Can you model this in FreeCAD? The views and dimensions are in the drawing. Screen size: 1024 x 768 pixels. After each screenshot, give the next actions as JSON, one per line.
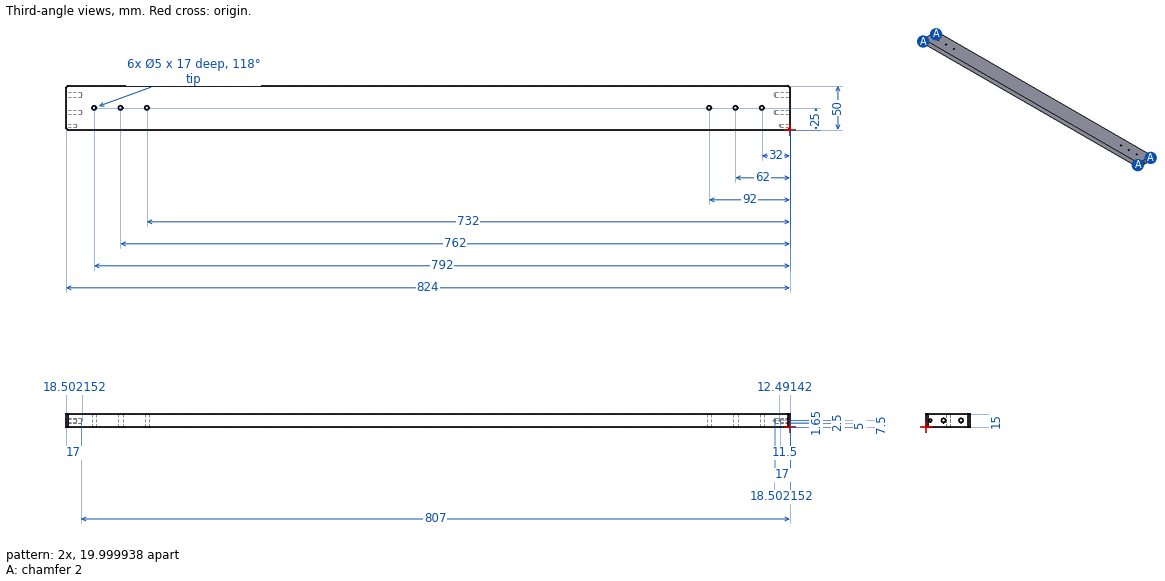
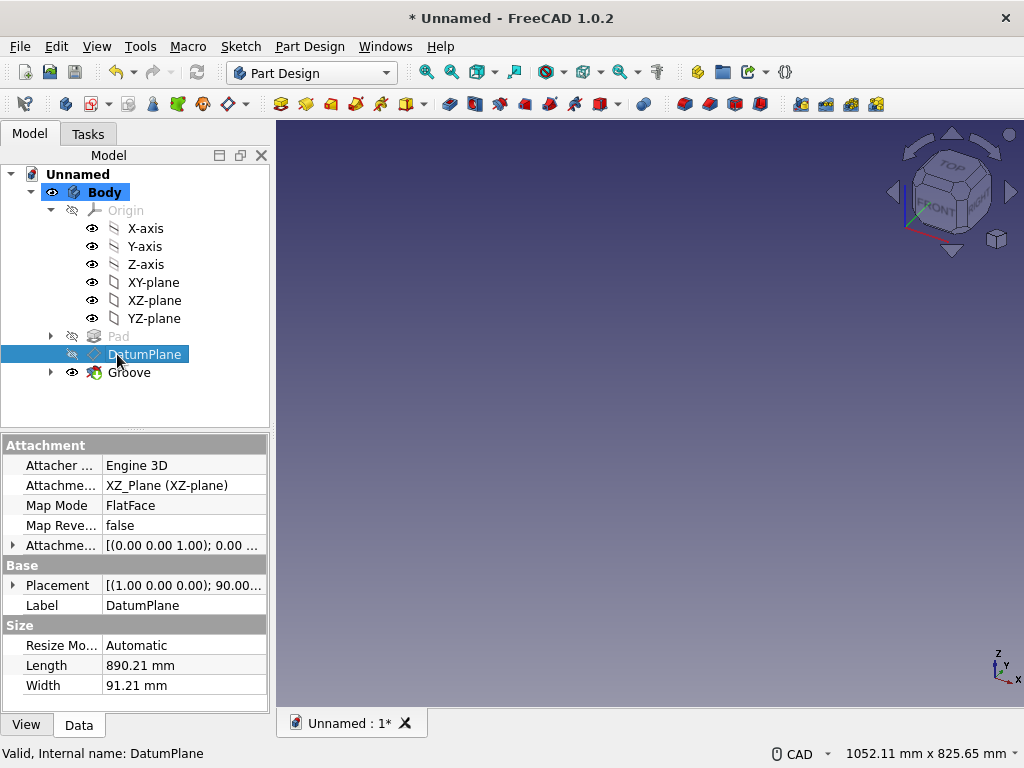
{"action": "left_click", "coordinate": [427, 72]}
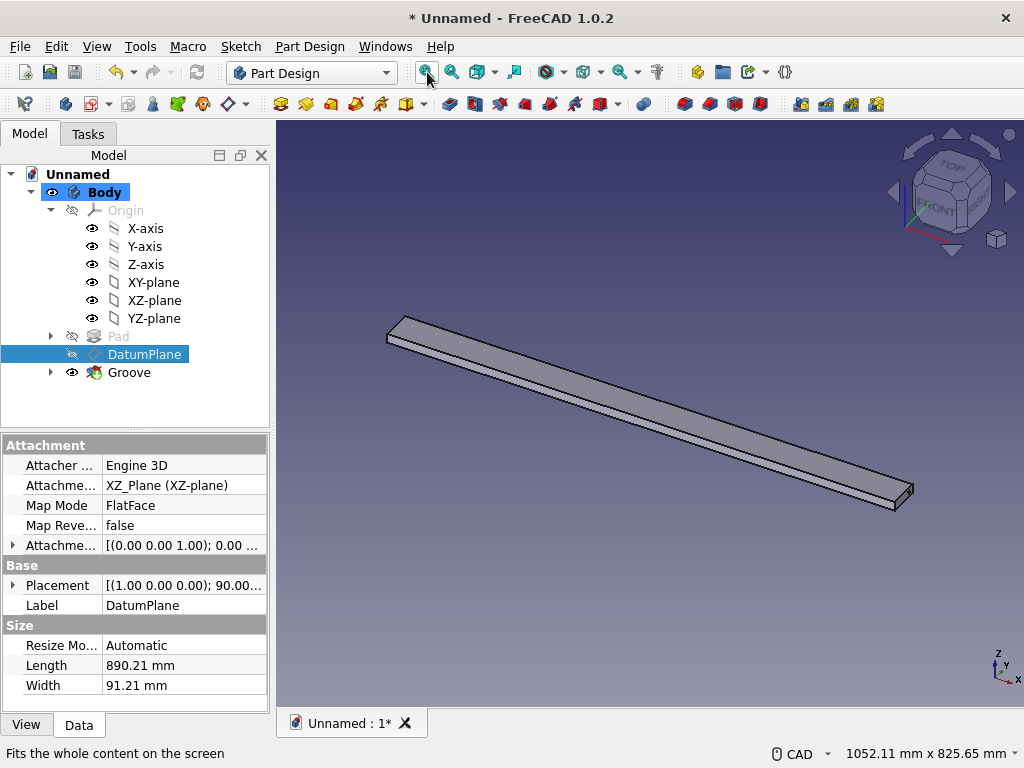
{"action": "left_click", "coordinate": [117, 372]}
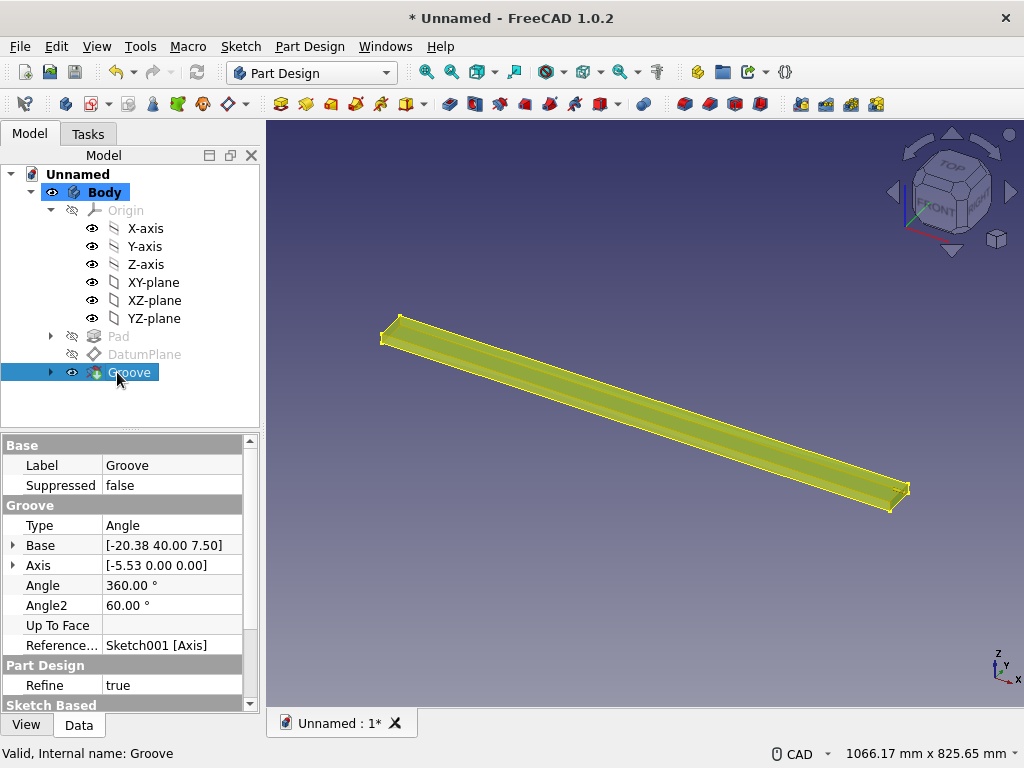
{"action": "left_click", "coordinate": [826, 104]}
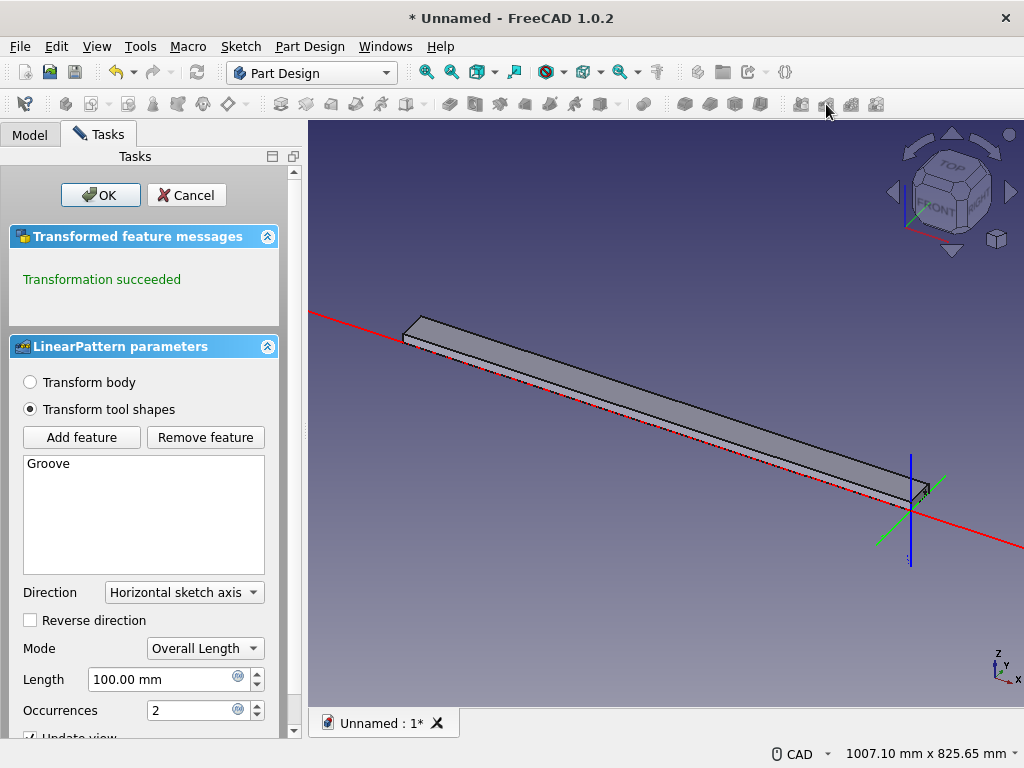
{"action": "left_click", "coordinate": [185, 592]}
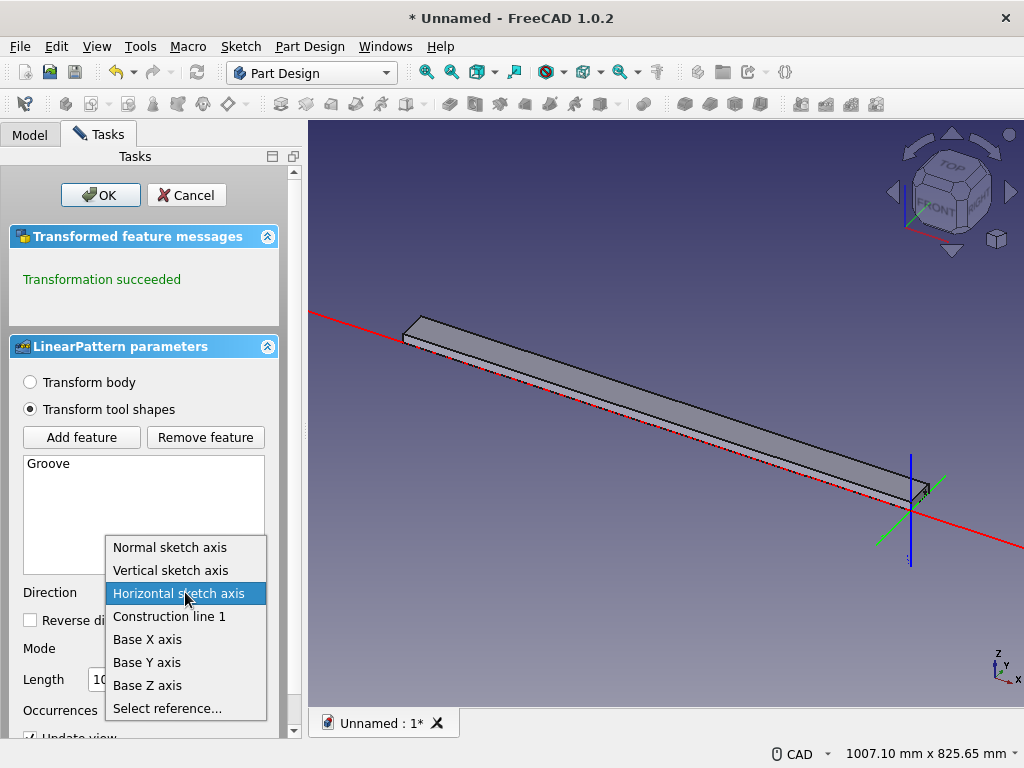
{"action": "left_click", "coordinate": [184, 662]}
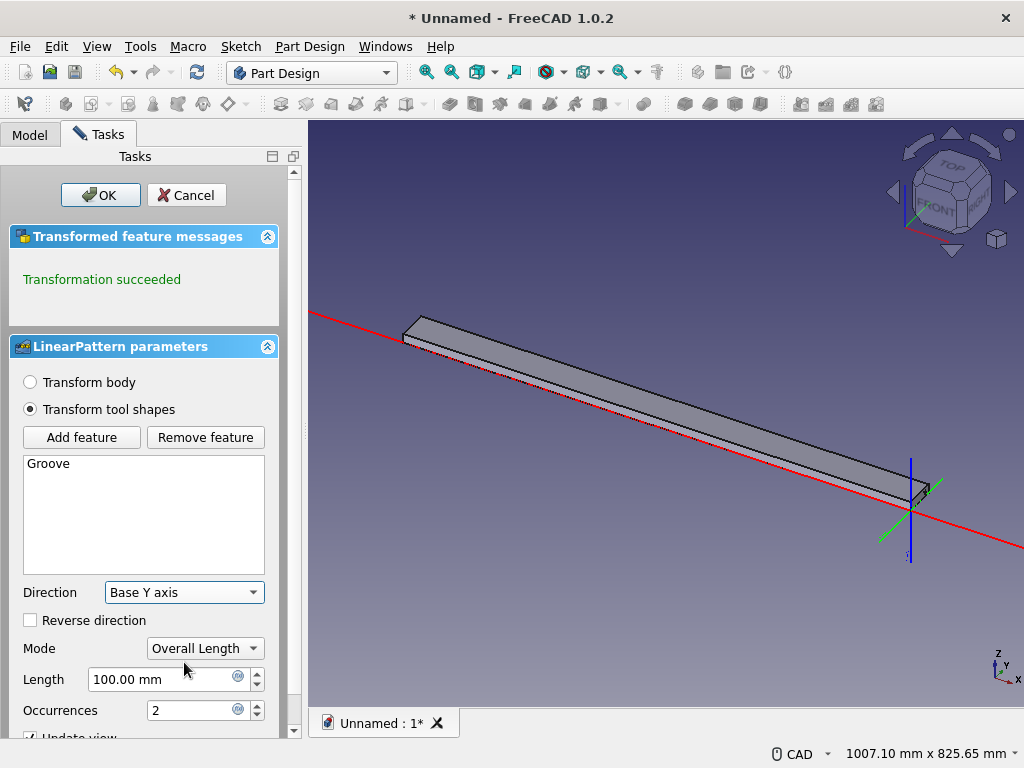
{"action": "left_click", "coordinate": [206, 648]}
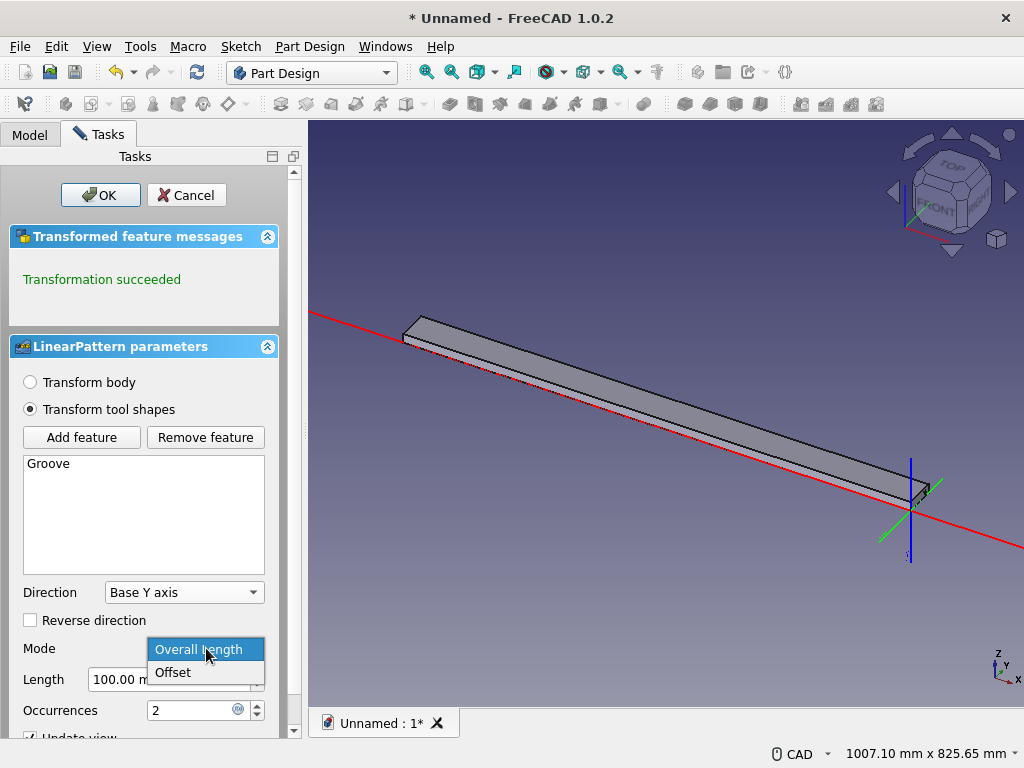
{"action": "left_click", "coordinate": [204, 672]}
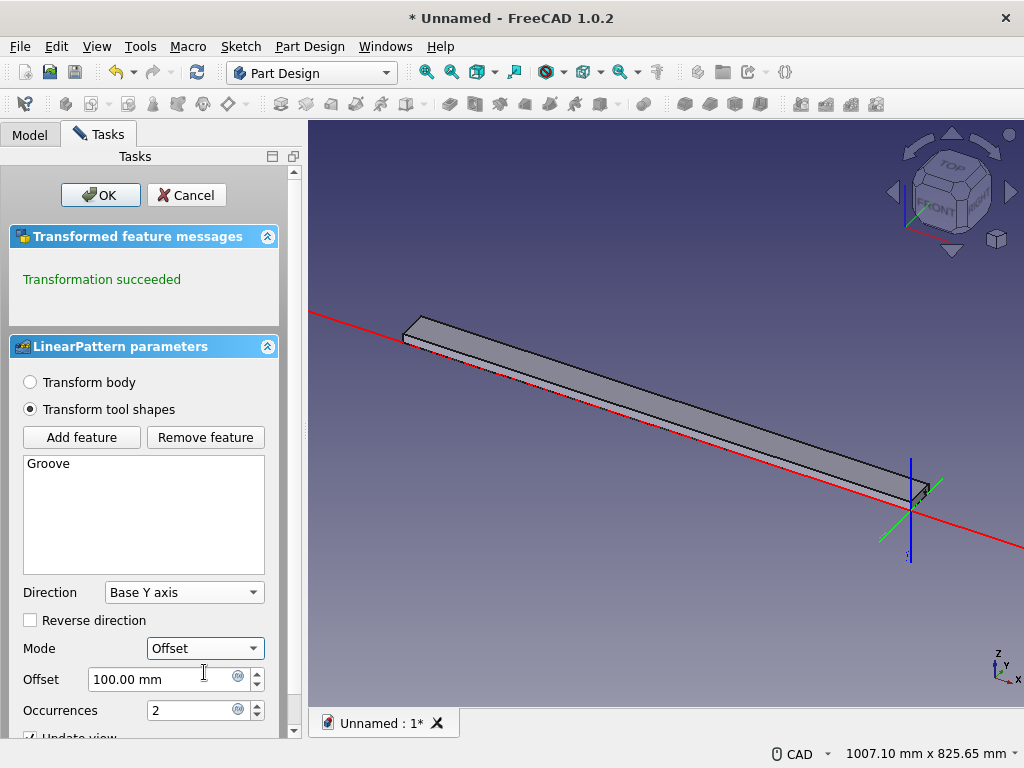
{"action": "triple_click", "coordinate": [170, 680]}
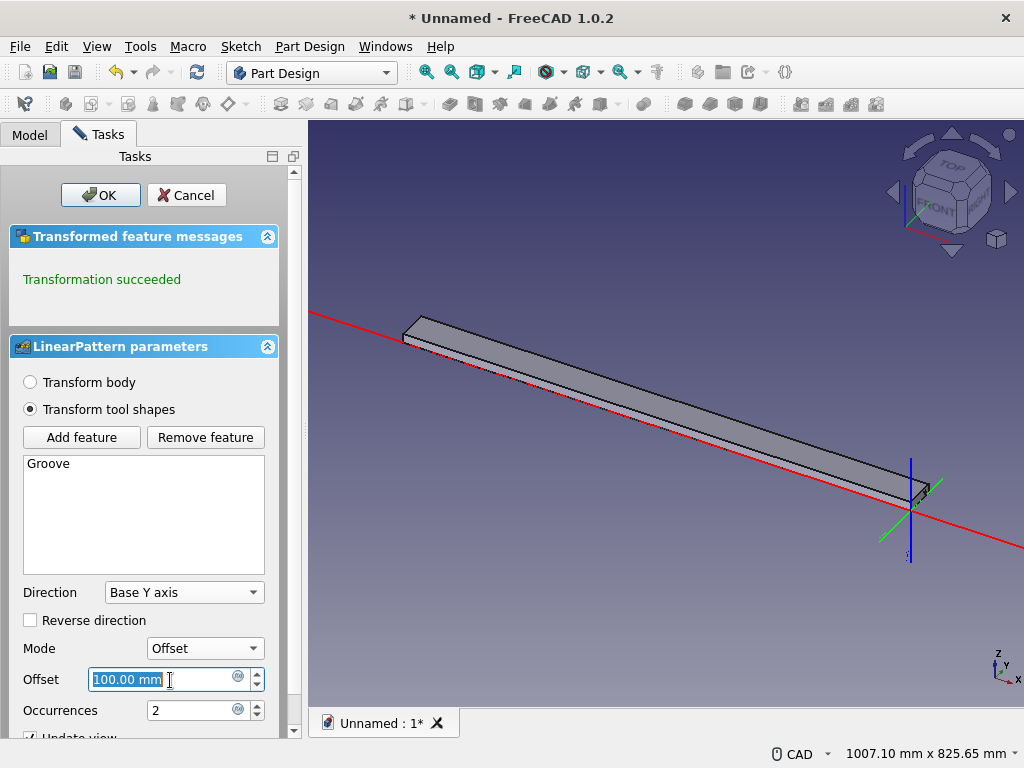
{"action": "type", "text": "19.999938"}
{"action": "key", "text": "Tab"}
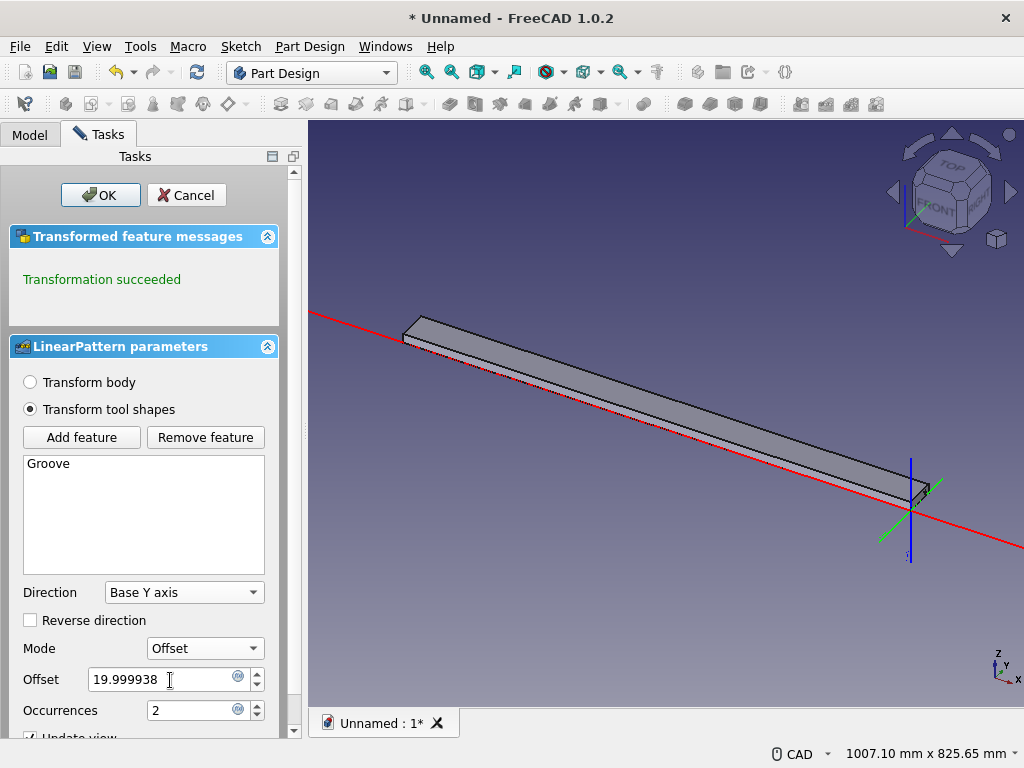
{"action": "triple_click", "coordinate": [199, 710]}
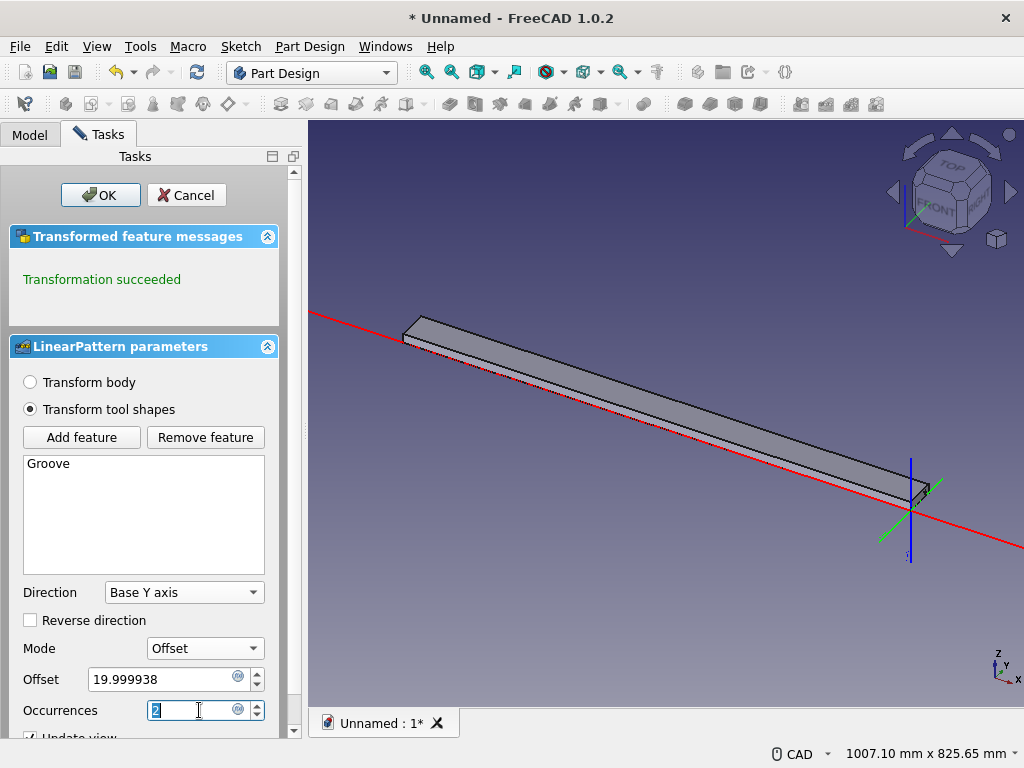
{"action": "type", "text": "2"}
{"action": "key", "text": "Tab"}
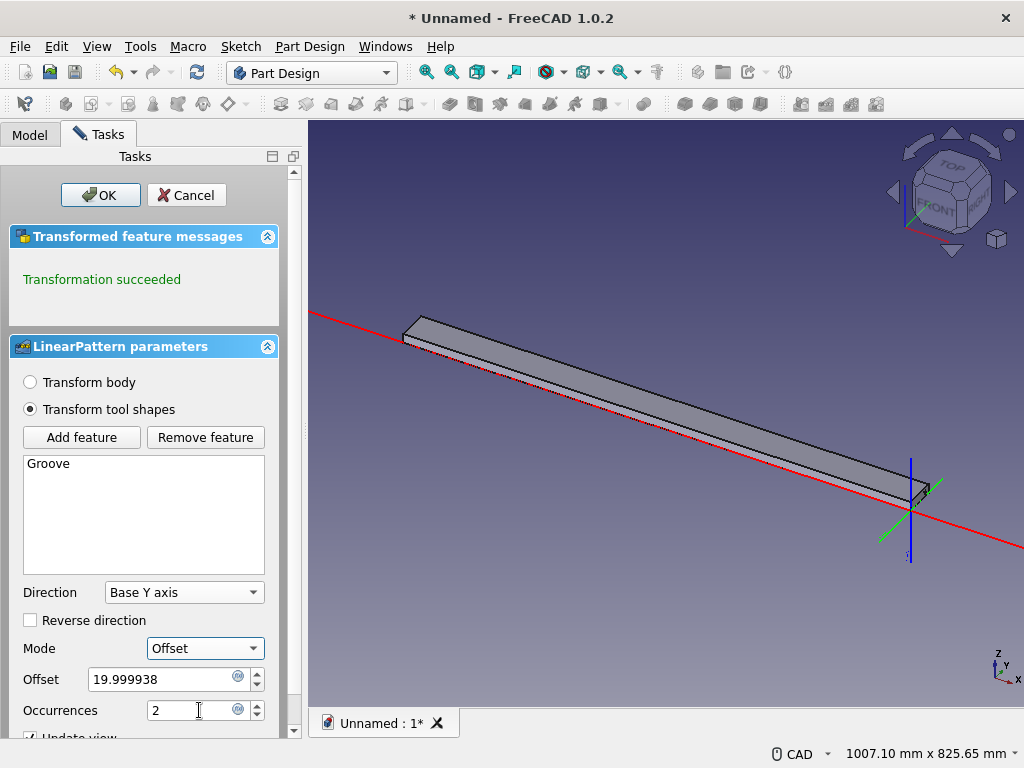
{"action": "left_click", "coordinate": [31, 620]}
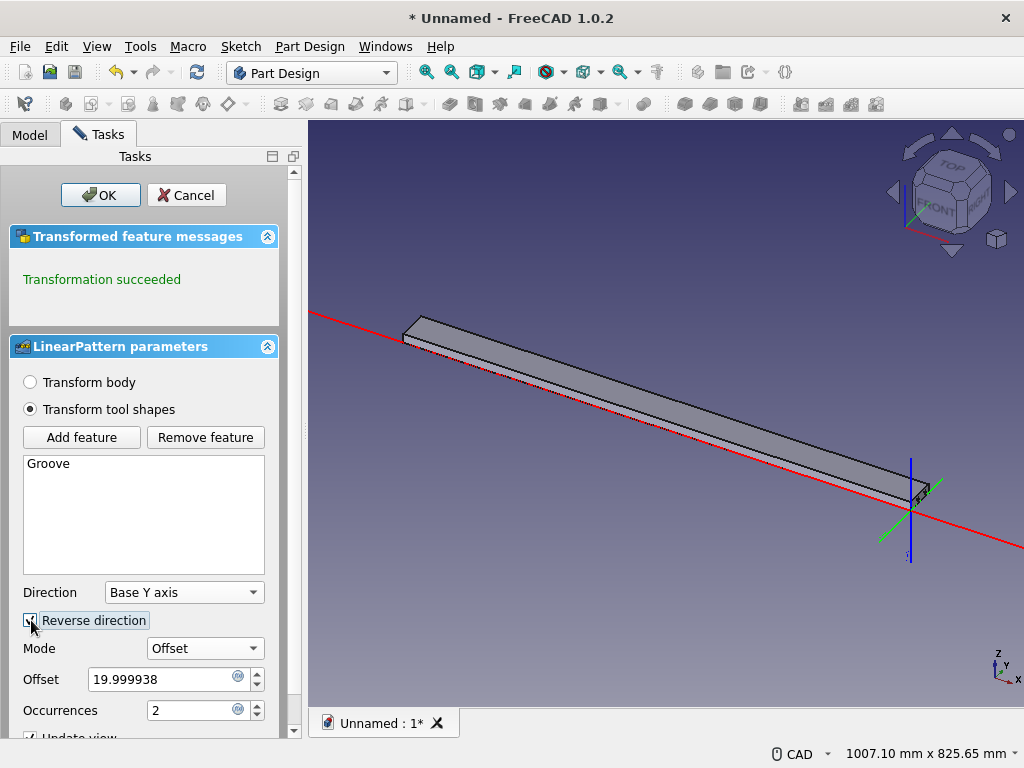
{"action": "left_click", "coordinate": [101, 195]}